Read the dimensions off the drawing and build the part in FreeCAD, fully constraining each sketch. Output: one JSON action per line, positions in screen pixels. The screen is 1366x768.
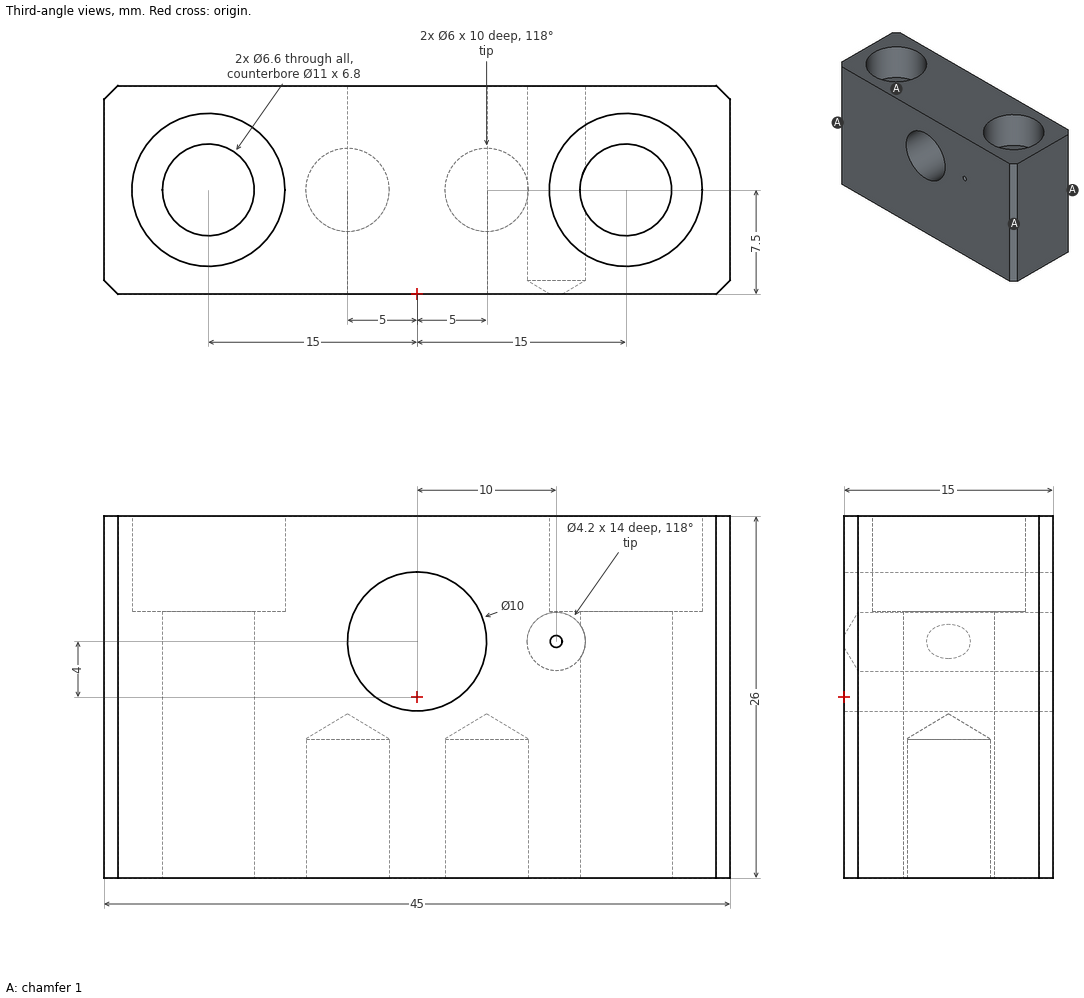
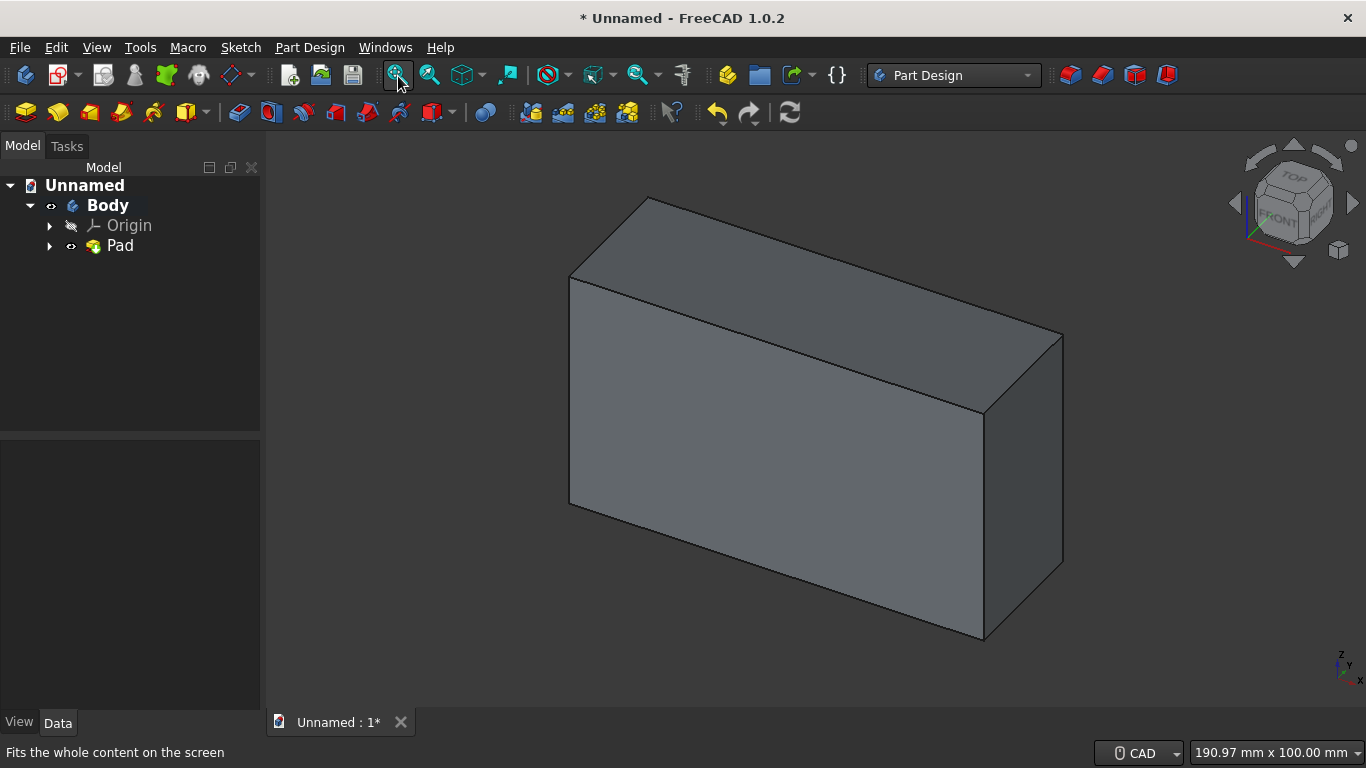
{"action": "key", "text": "4"}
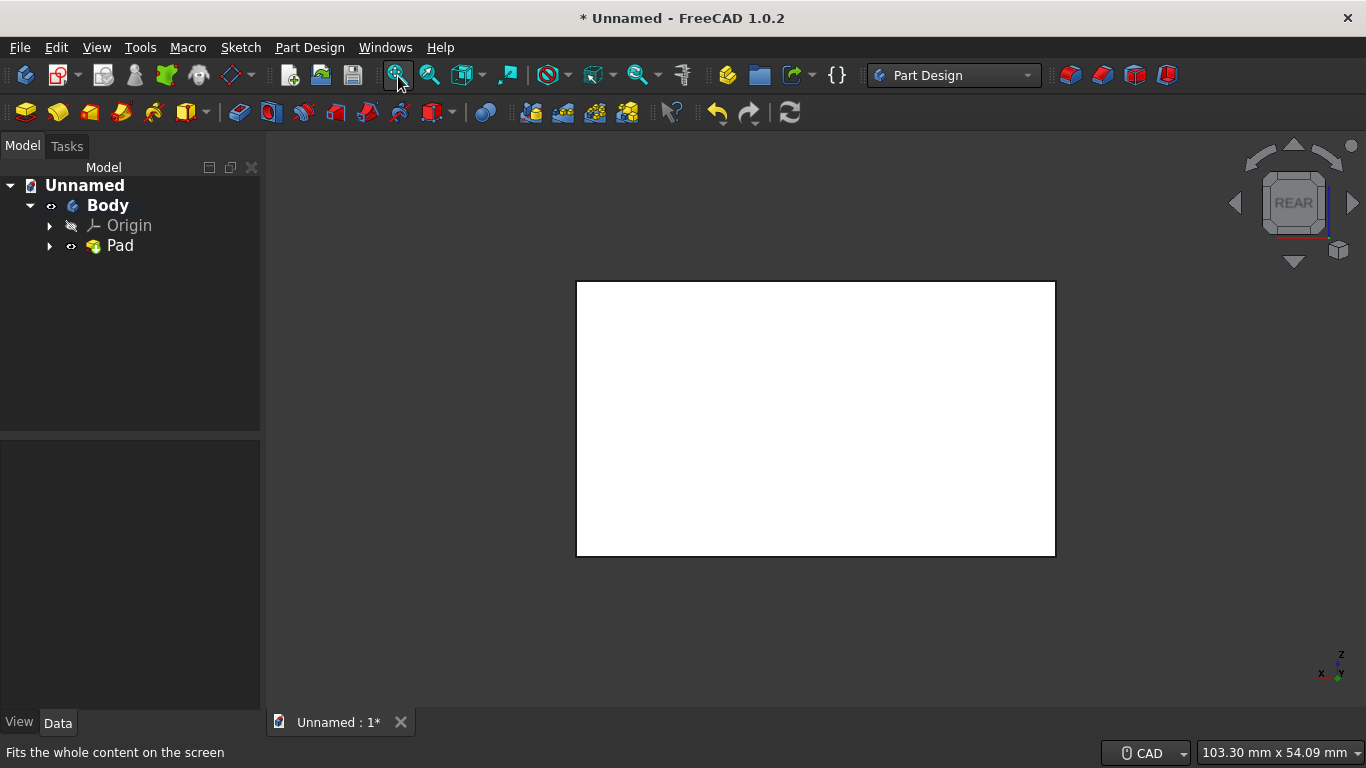
{"action": "left_click", "coordinate": [748, 418]}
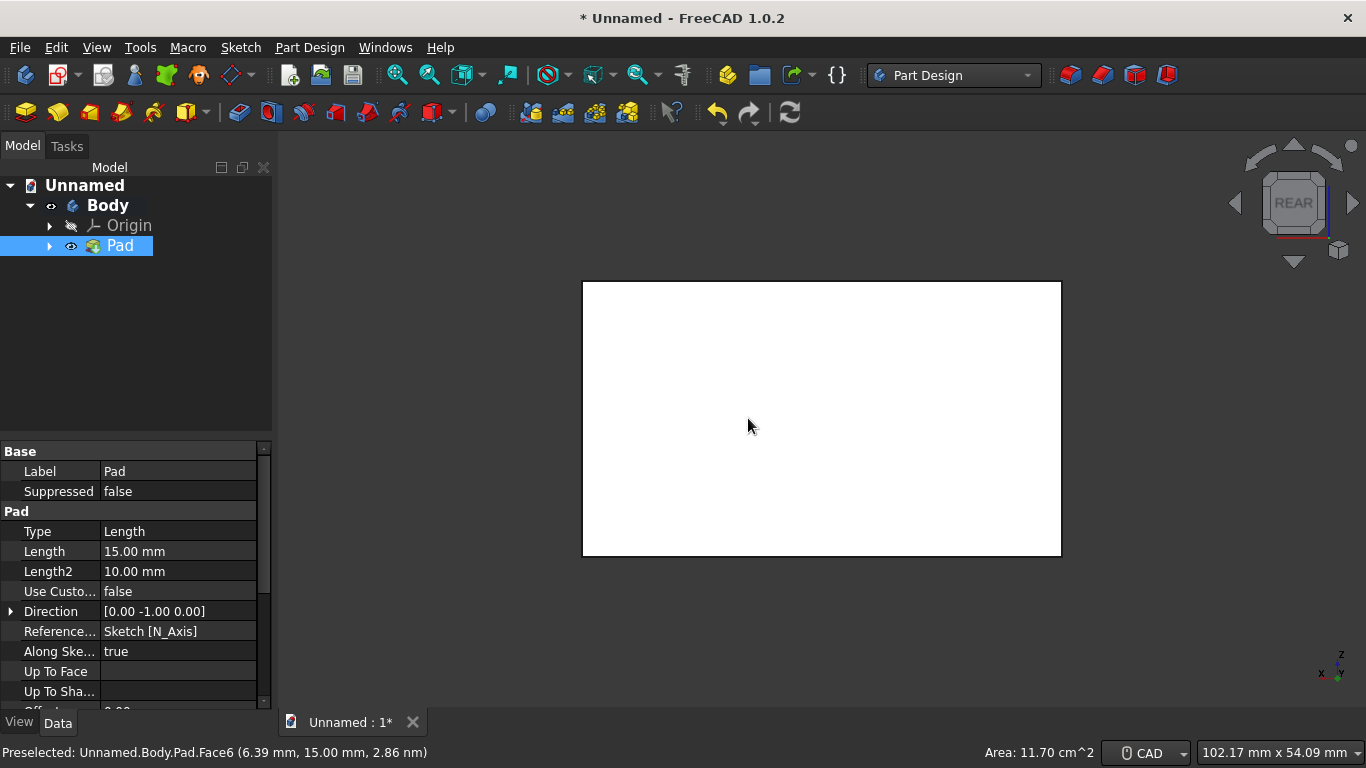
{"action": "left_click", "coordinate": [58, 76]}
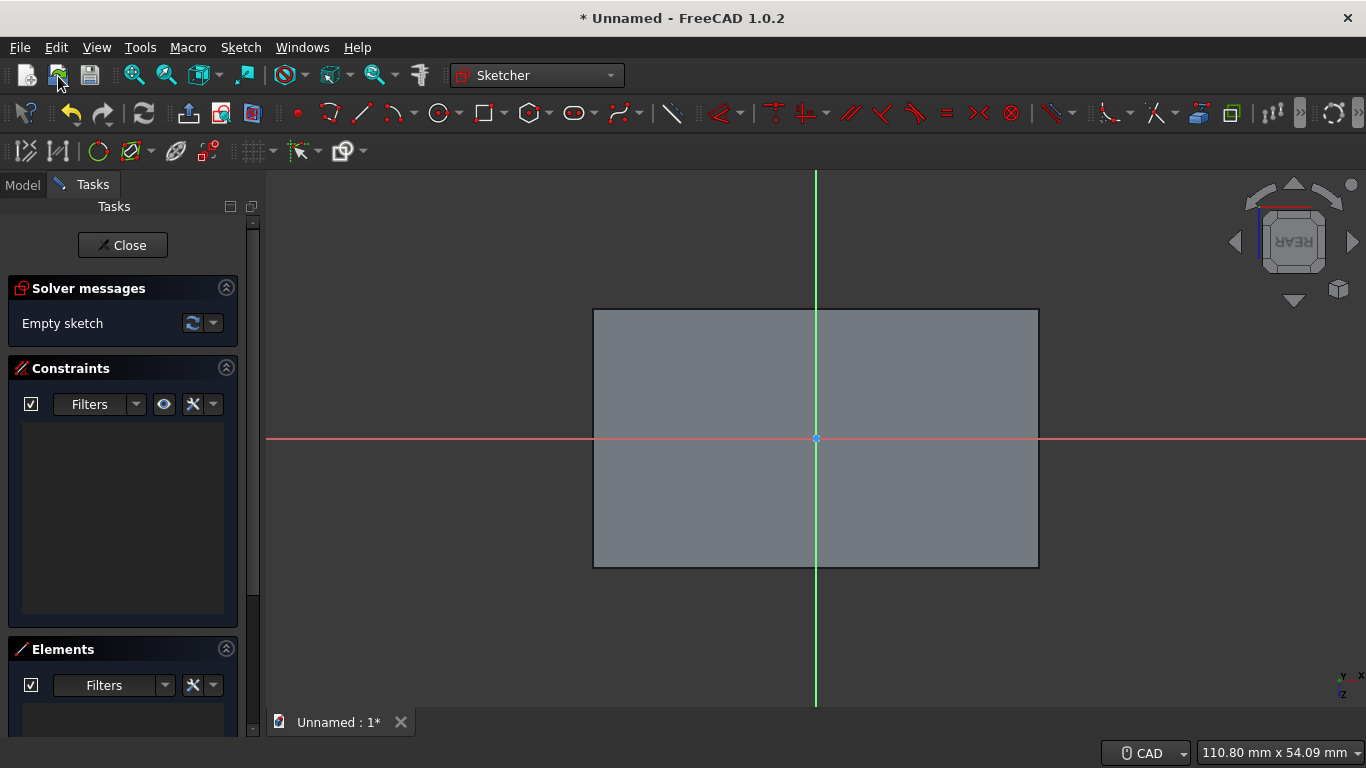
{"action": "scroll", "coordinate": [846, 495], "scroll_direction": "up", "scroll_amount": 6}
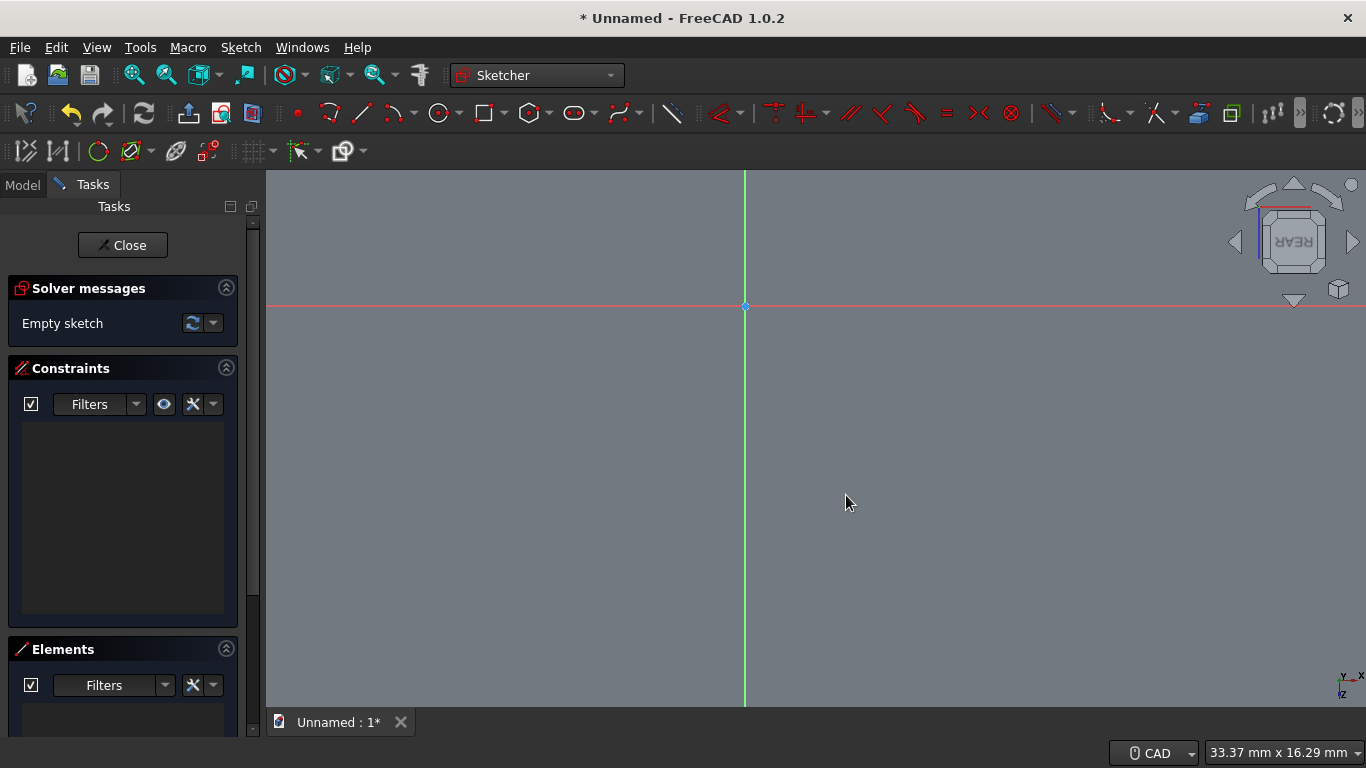
{"action": "left_click", "coordinate": [440, 114]}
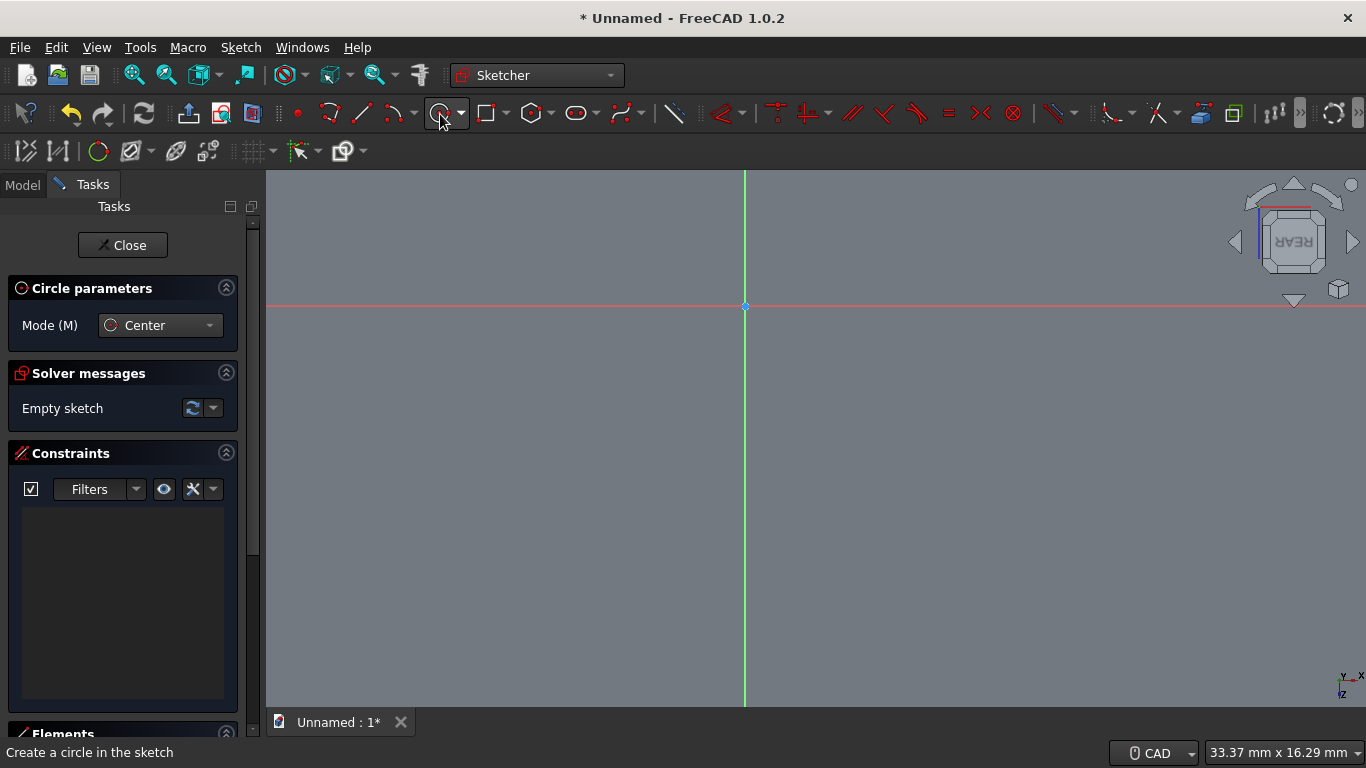
{"action": "left_click", "coordinate": [745, 438]}
{"action": "left_click", "coordinate": [862, 321]}
{"action": "key", "text": "Escape"}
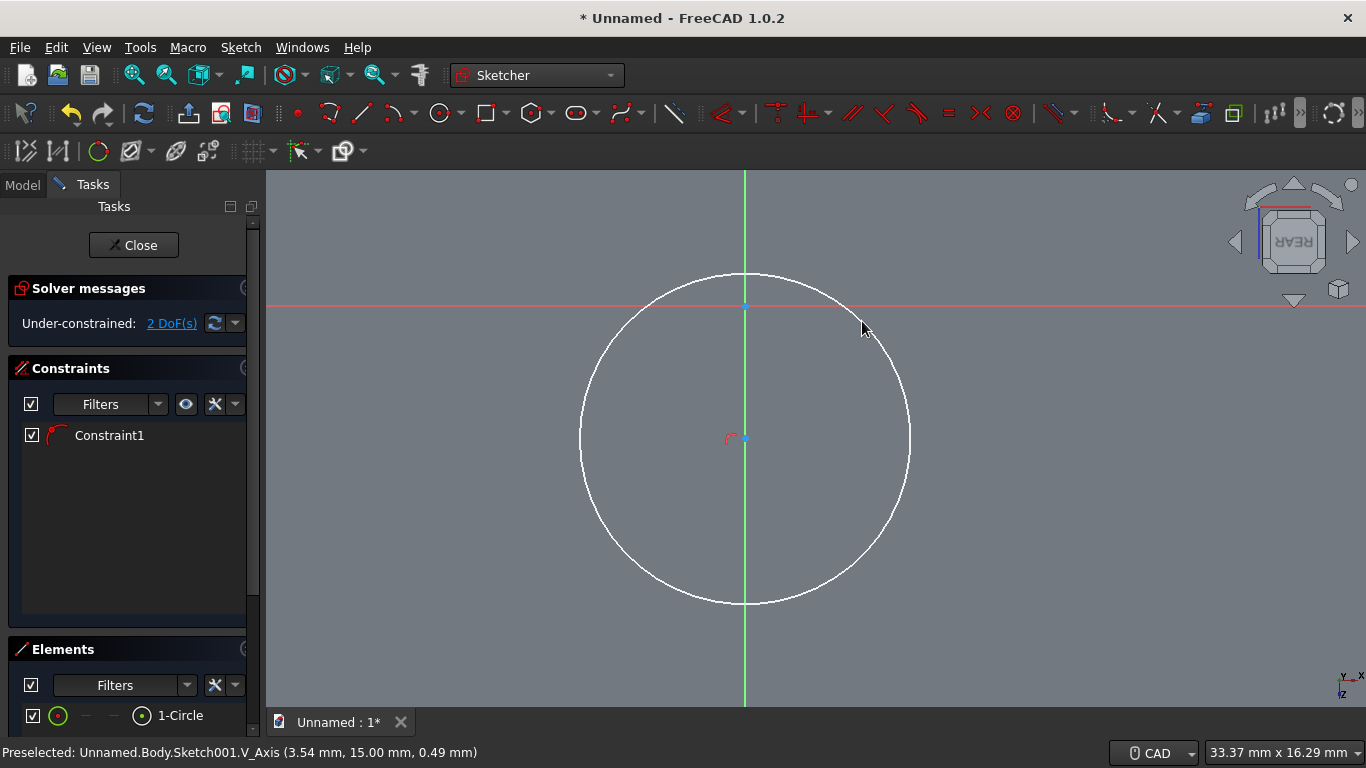
{"action": "left_click", "coordinate": [722, 114]}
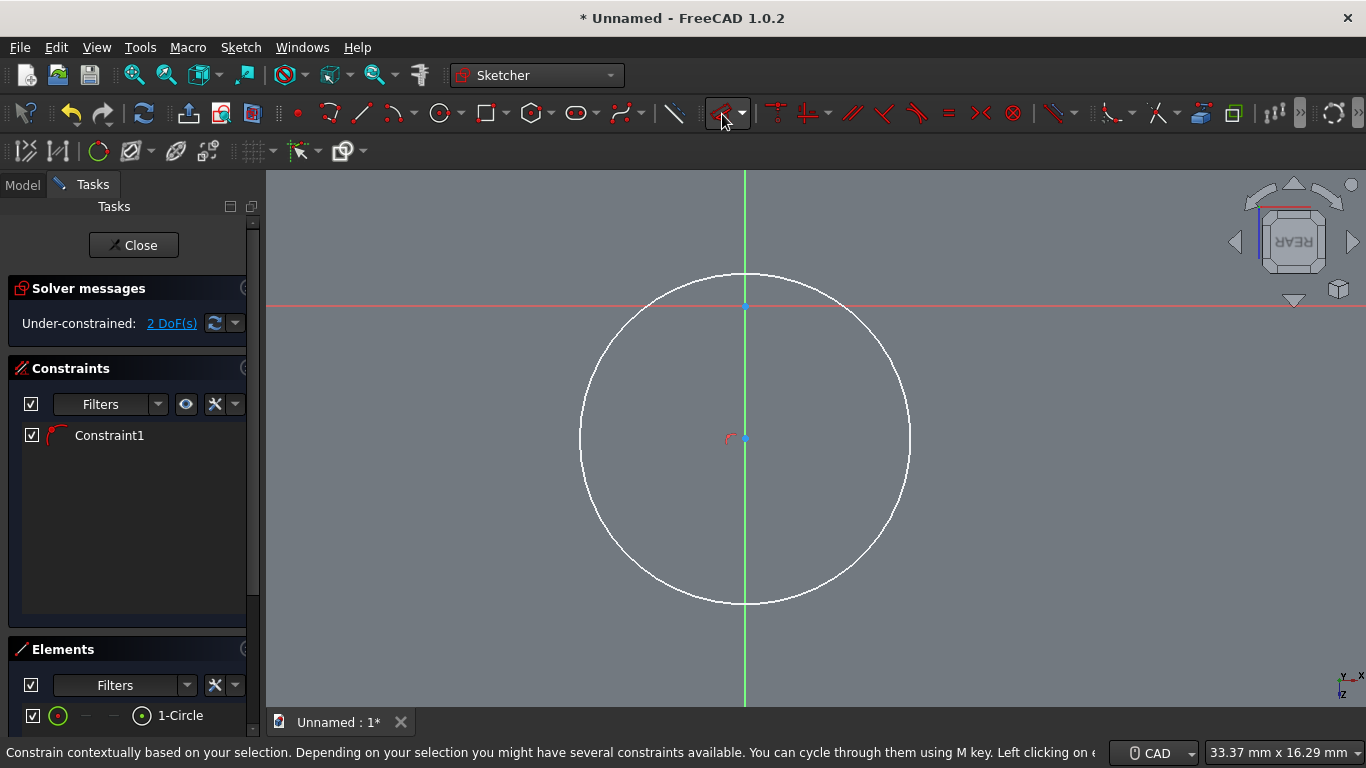
{"action": "left_click", "coordinate": [862, 322]}
{"action": "left_click", "coordinate": [934, 383]}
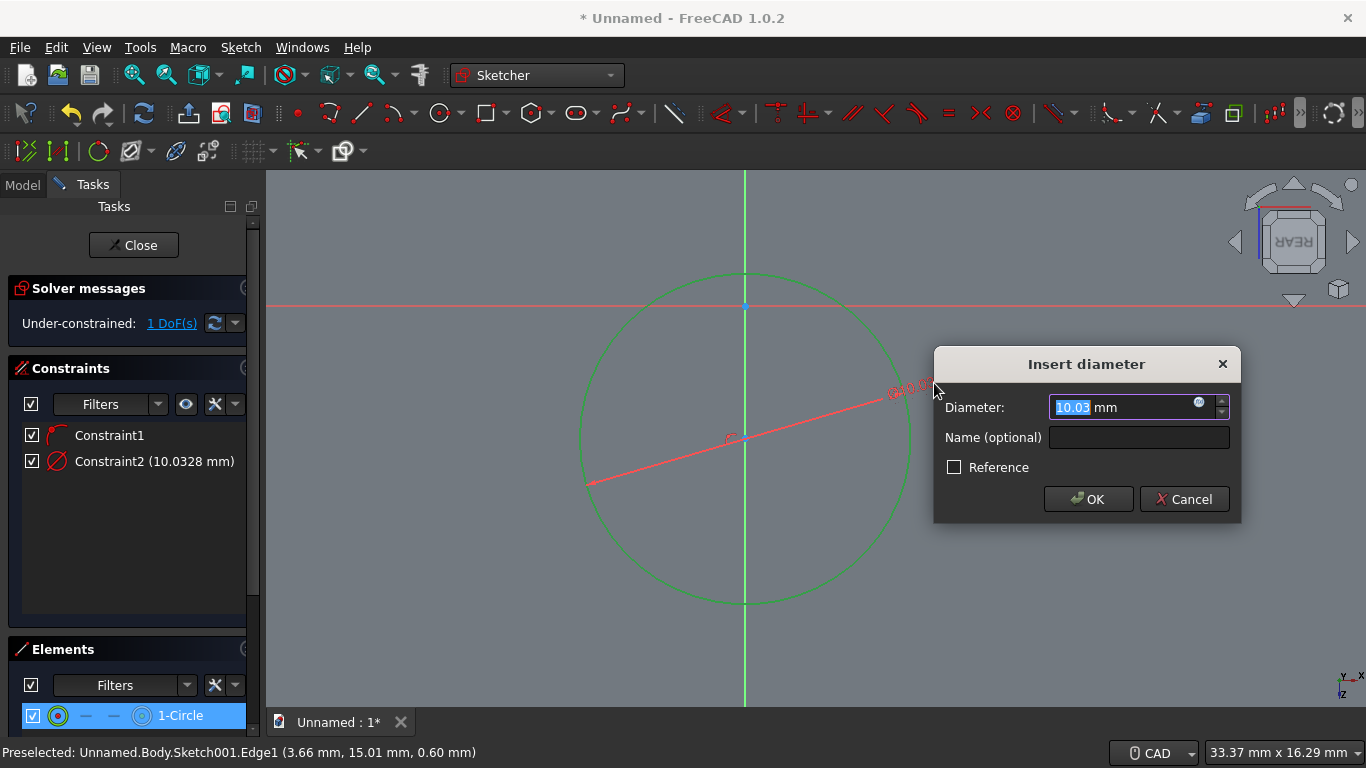
{"action": "type", "text": "10"}
{"action": "key", "text": "Return"}